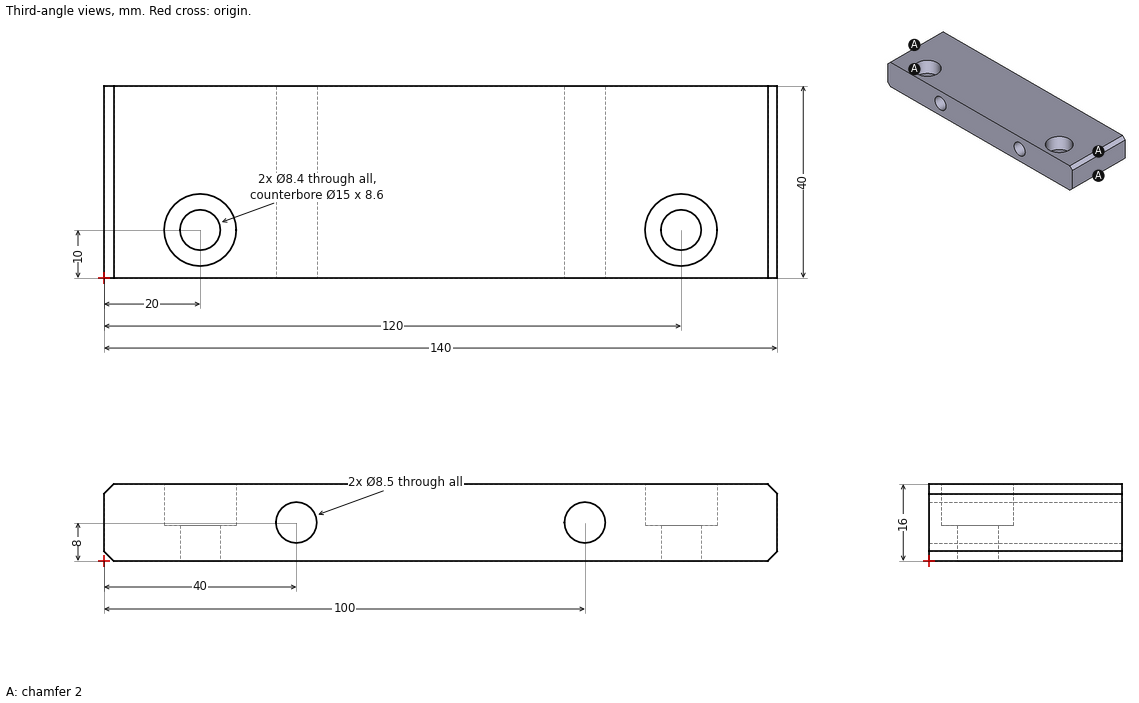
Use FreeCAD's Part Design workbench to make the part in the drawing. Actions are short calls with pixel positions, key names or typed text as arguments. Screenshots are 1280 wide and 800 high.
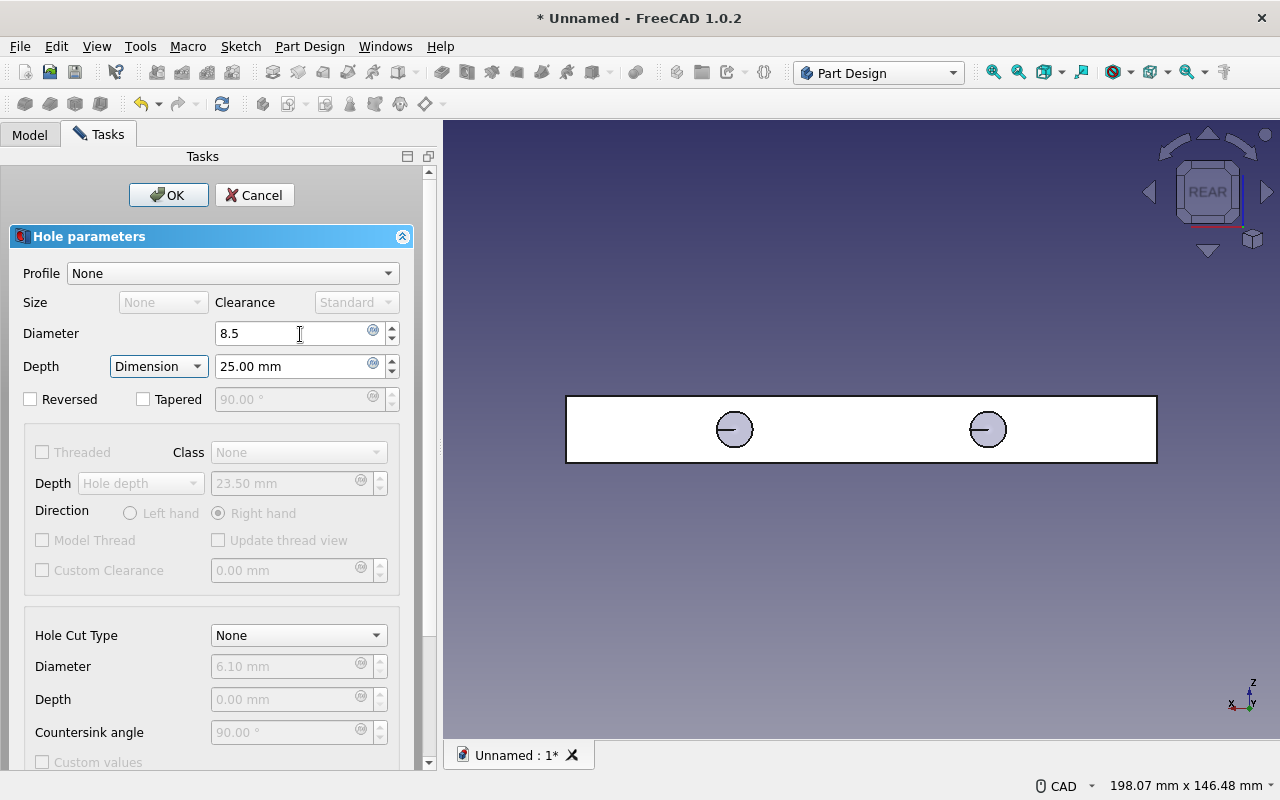
click(160, 366)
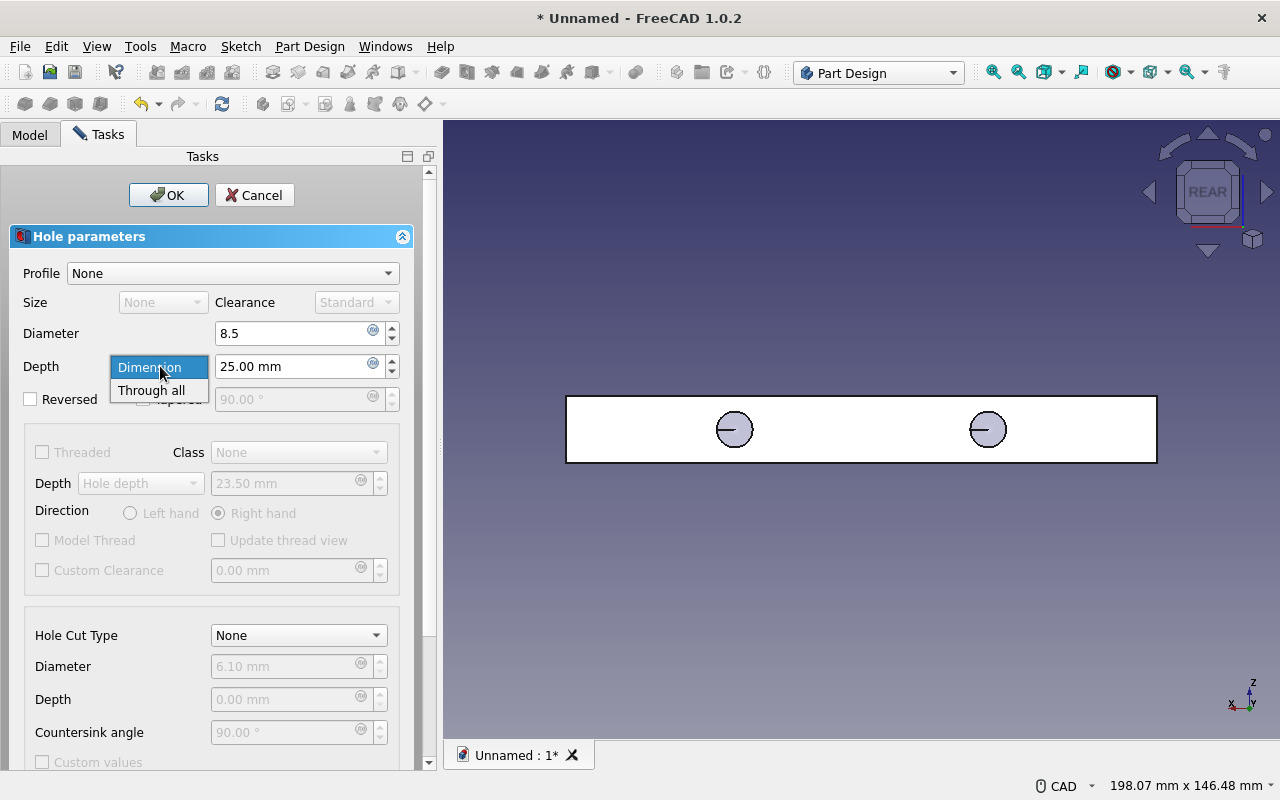
click(158, 390)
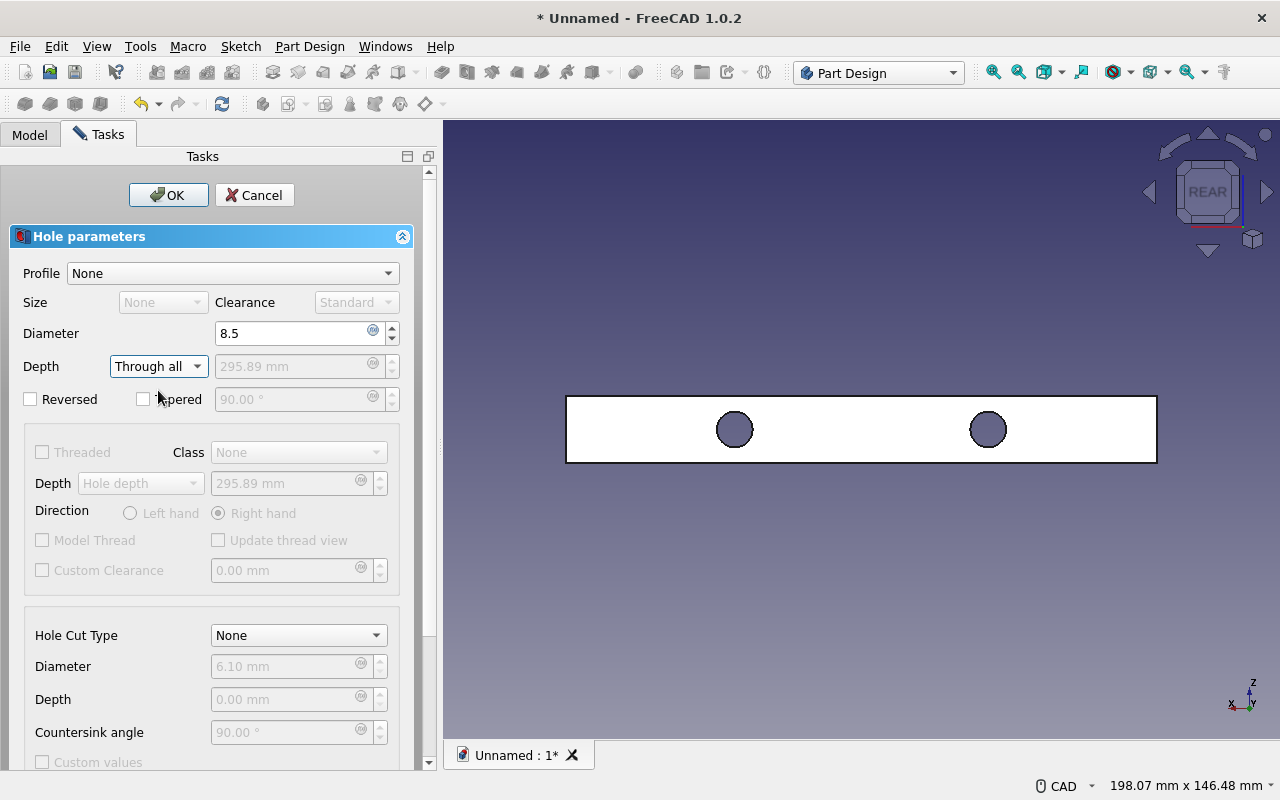
click(169, 195)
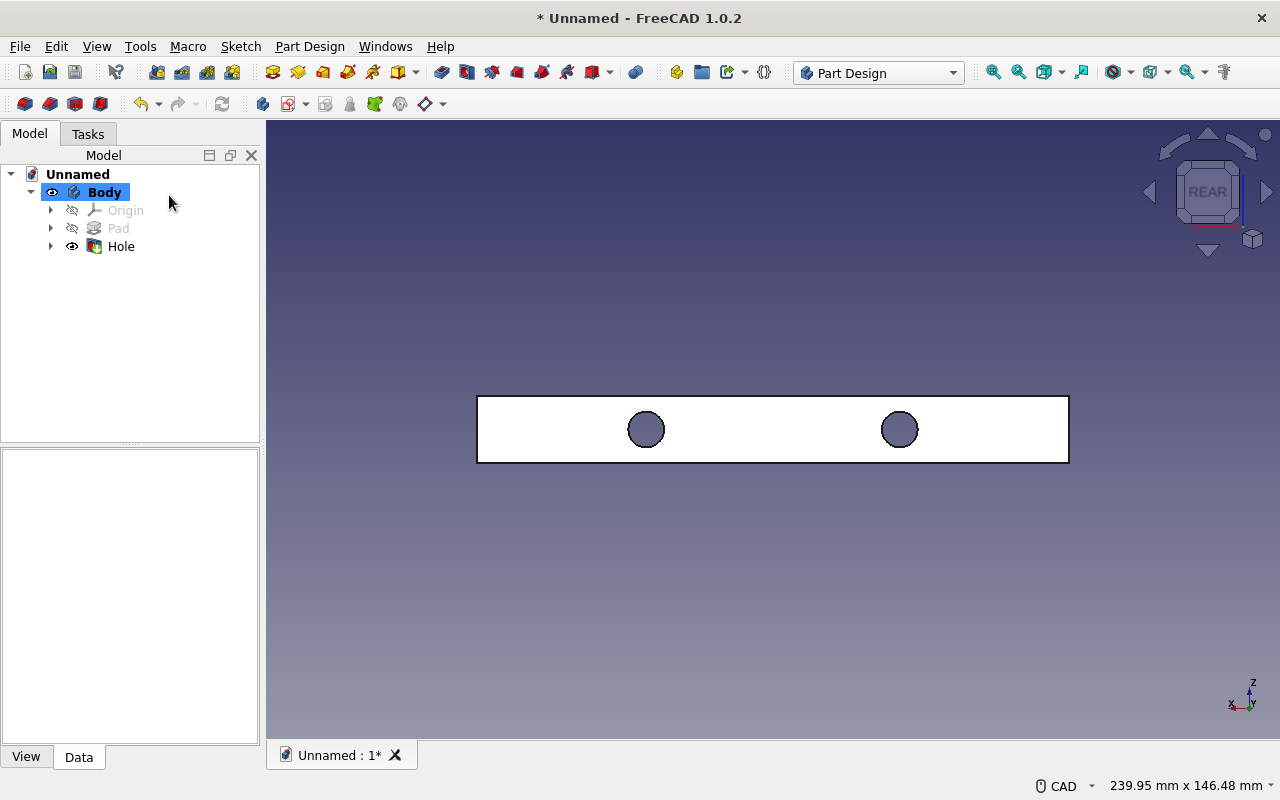
key(0)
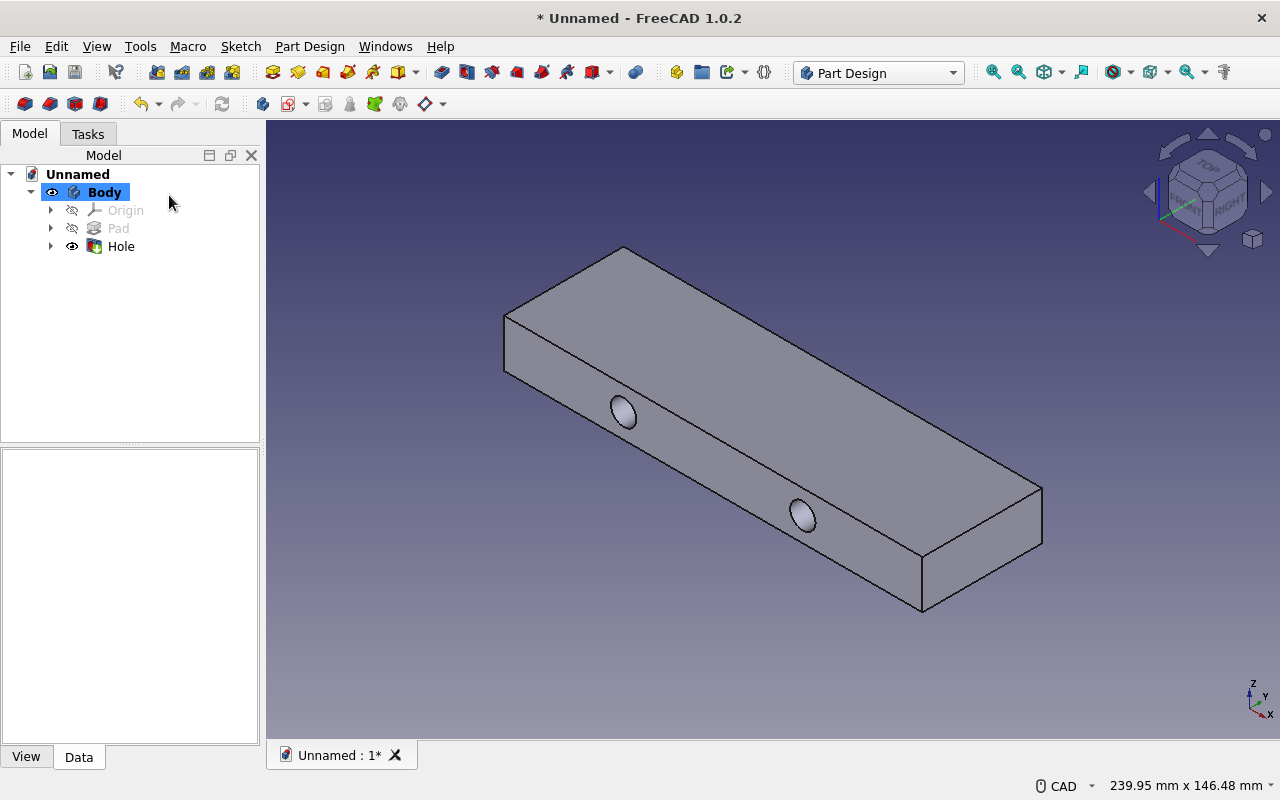
click(893, 470)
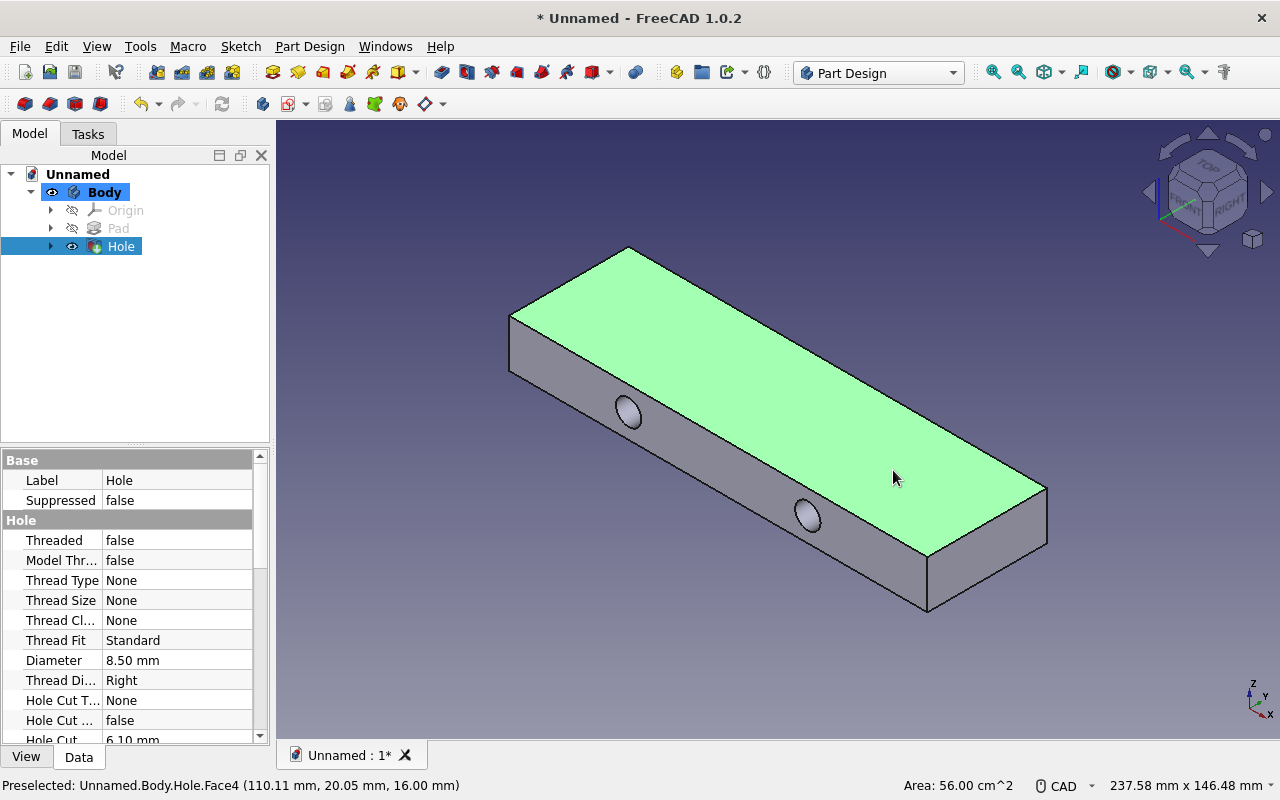
click(288, 104)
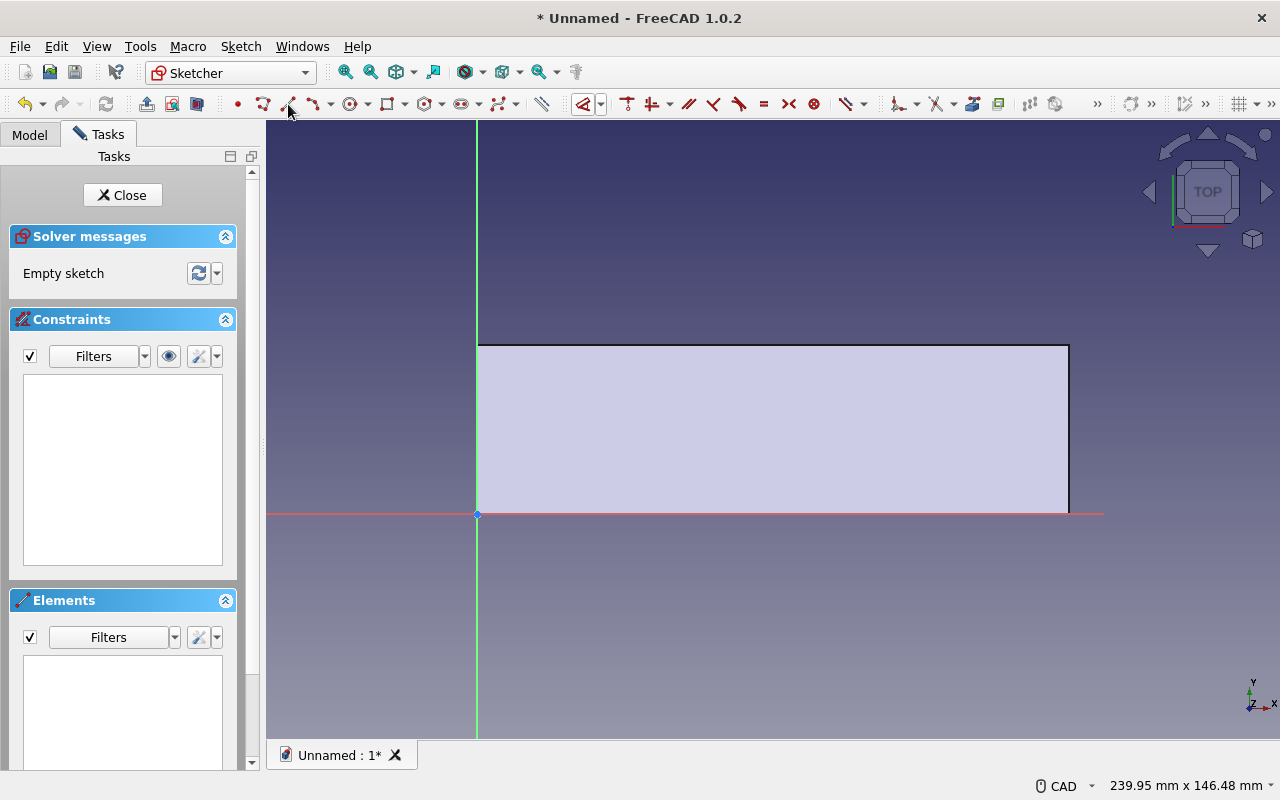
click(350, 104)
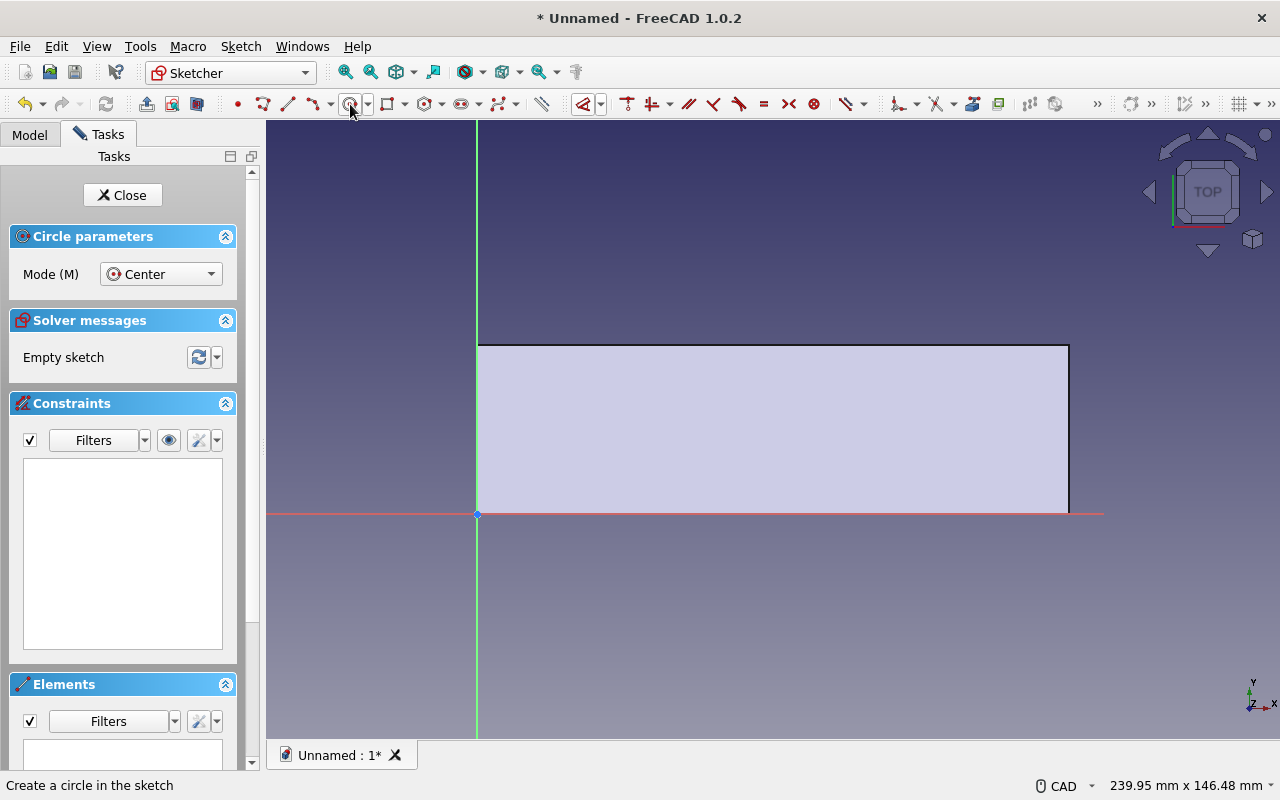
scroll(562, 472, up, 2)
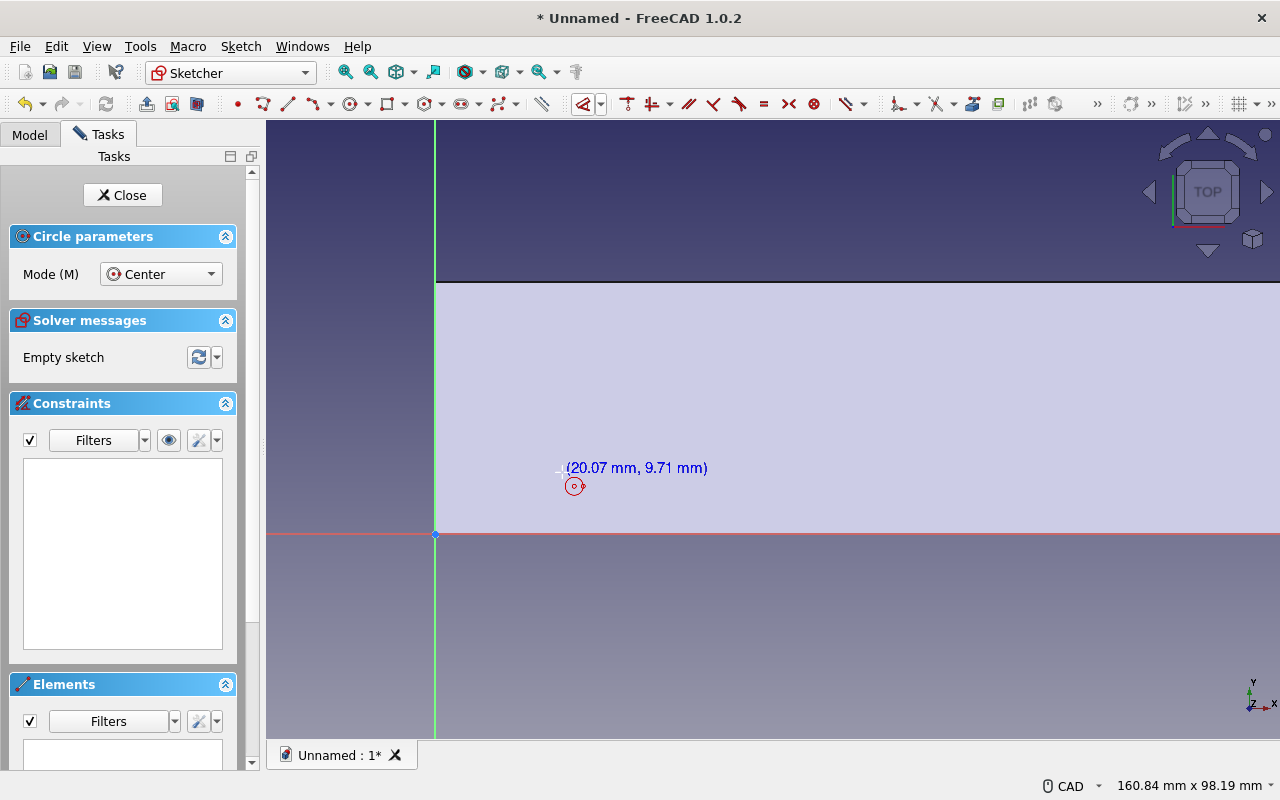
click(561, 471)
click(580, 453)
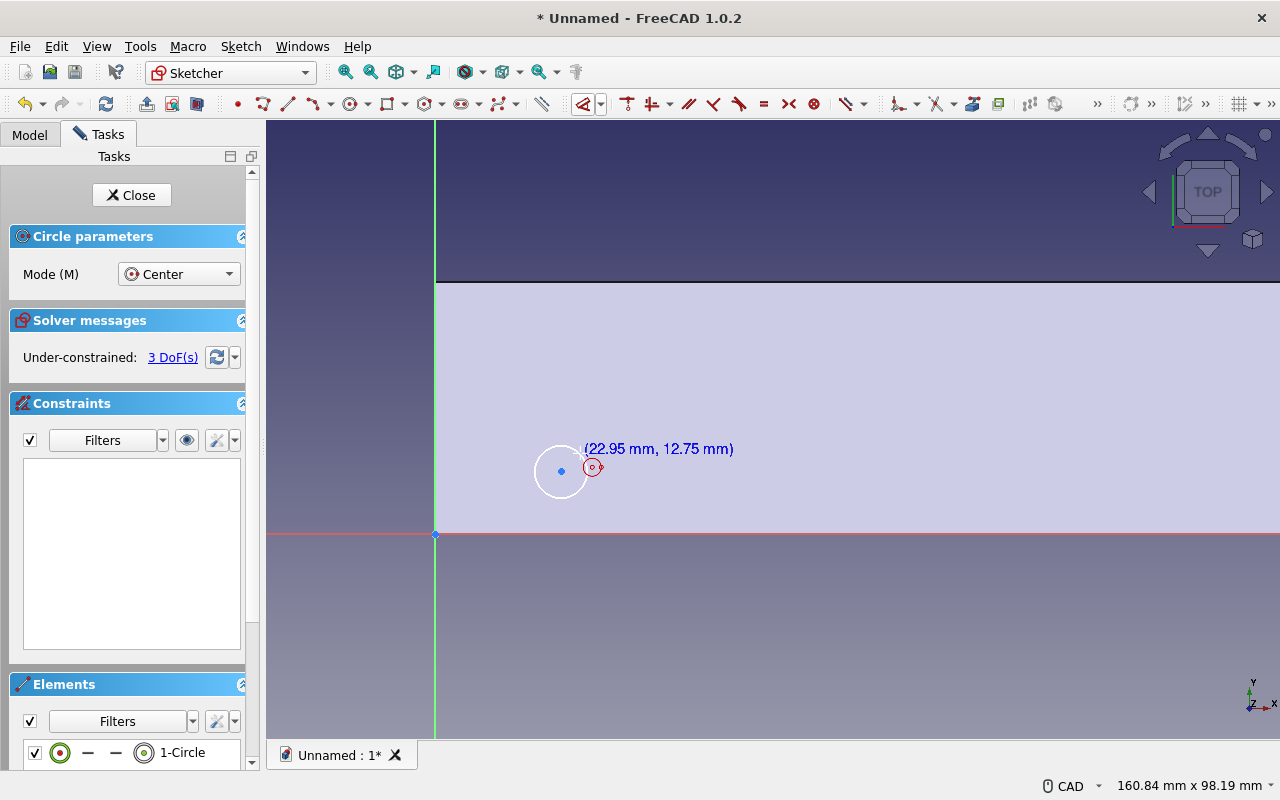
scroll(456, 307, down, 2)